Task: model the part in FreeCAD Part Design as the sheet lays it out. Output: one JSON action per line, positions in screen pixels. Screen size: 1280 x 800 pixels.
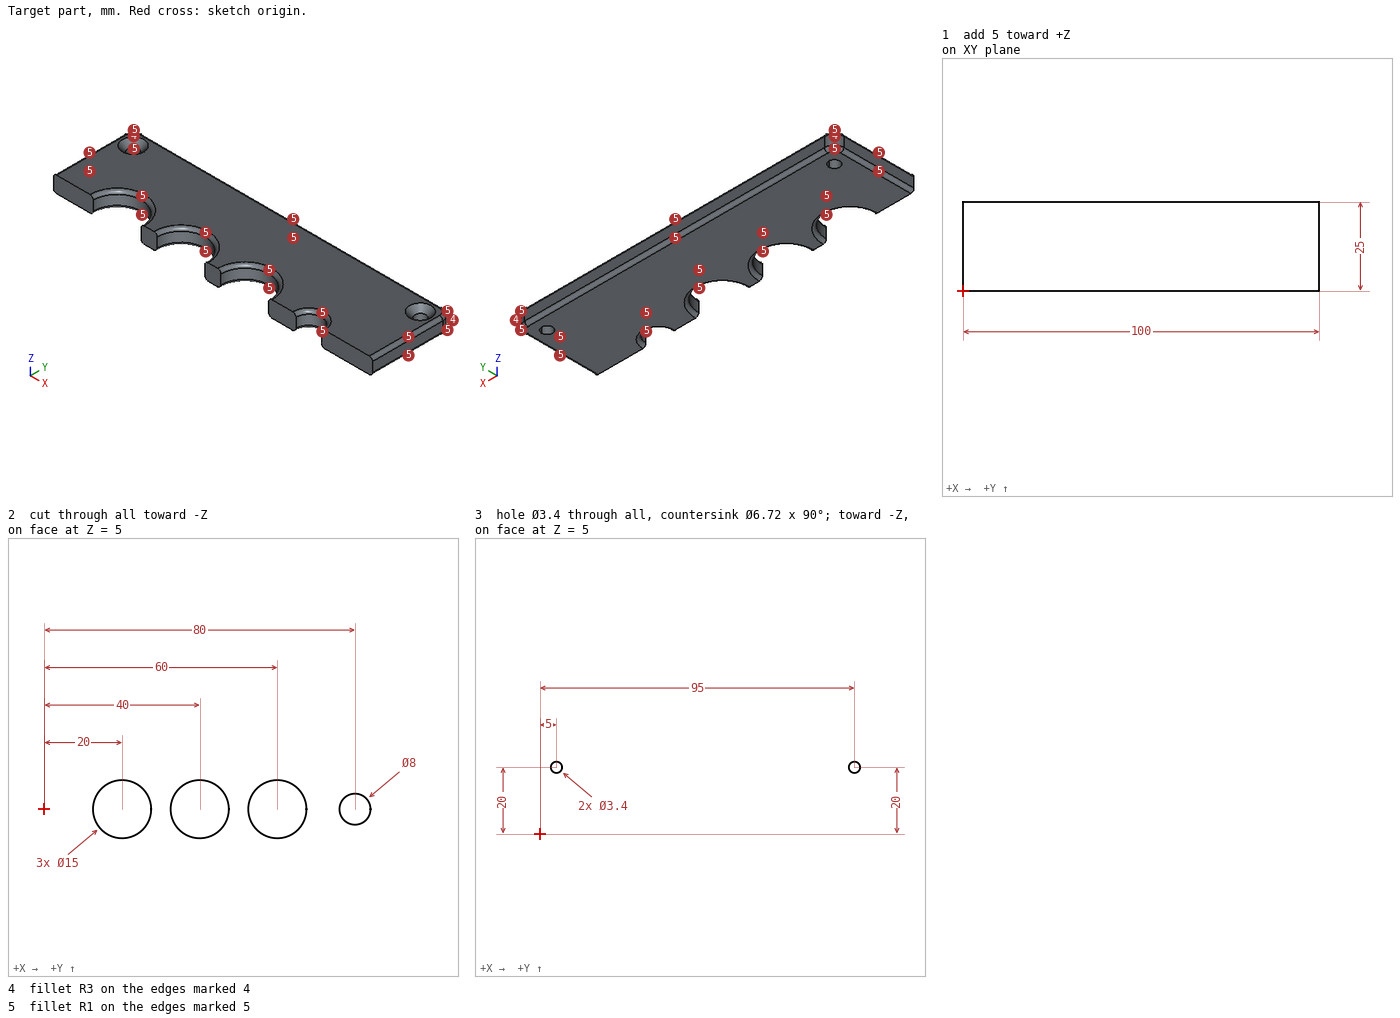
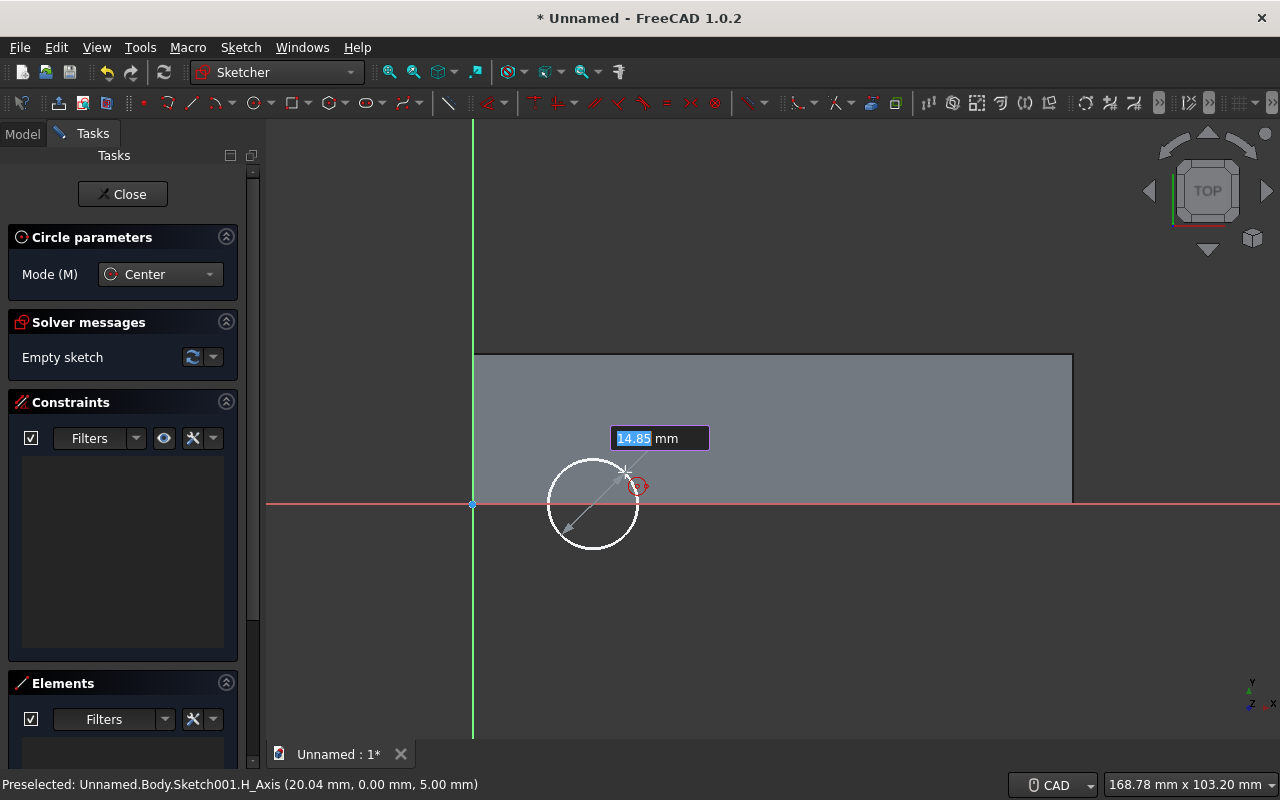
{"action": "type", "text": "15"}
{"action": "key", "text": "Return"}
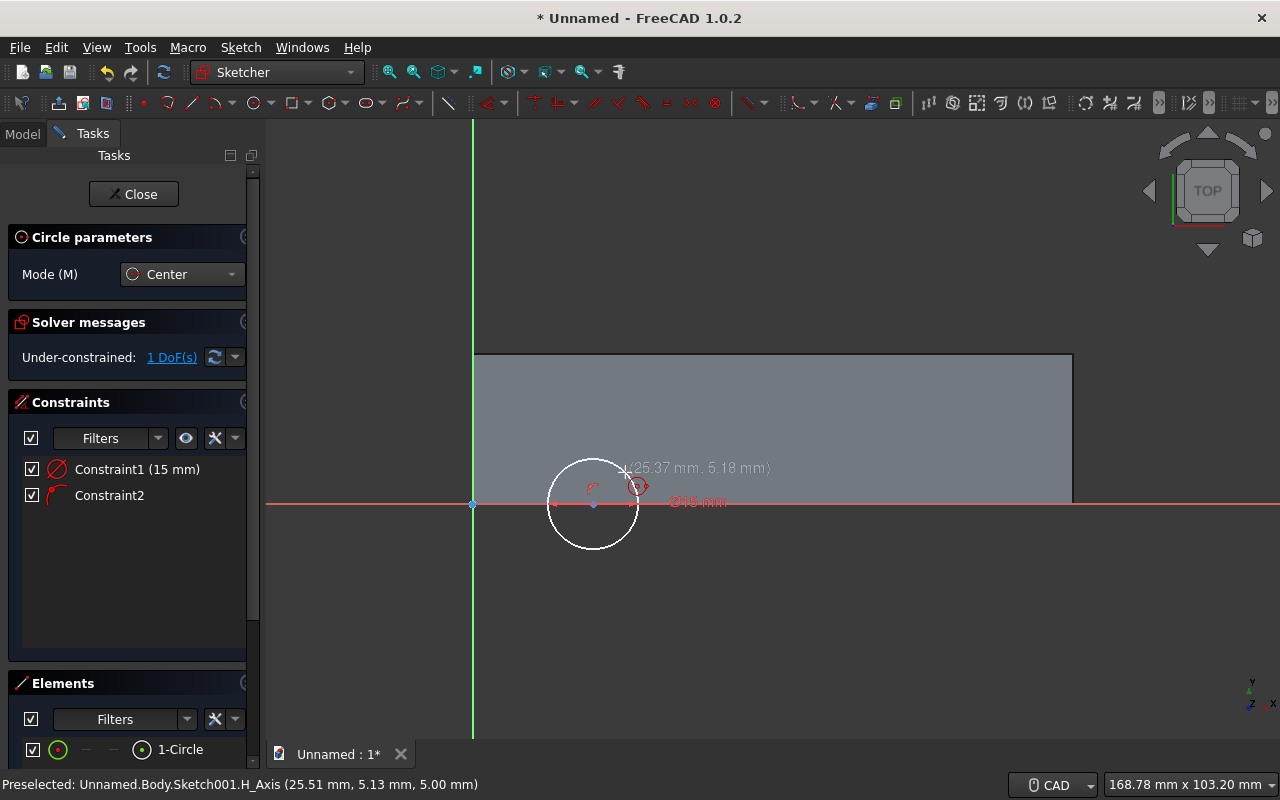
{"action": "left_click", "coordinate": [713, 504]}
{"action": "mouse_move", "coordinate": [745, 472]}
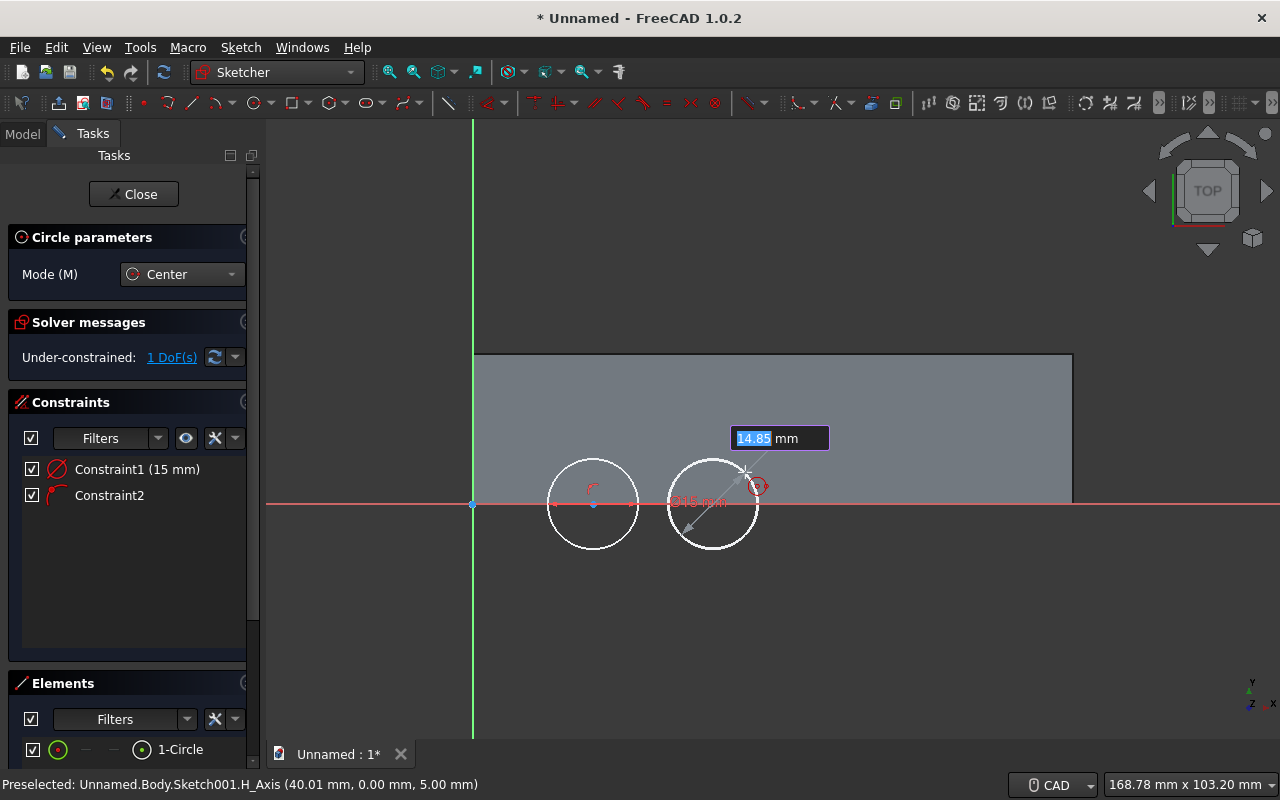
{"action": "type", "text": "15"}
{"action": "key", "text": "Return"}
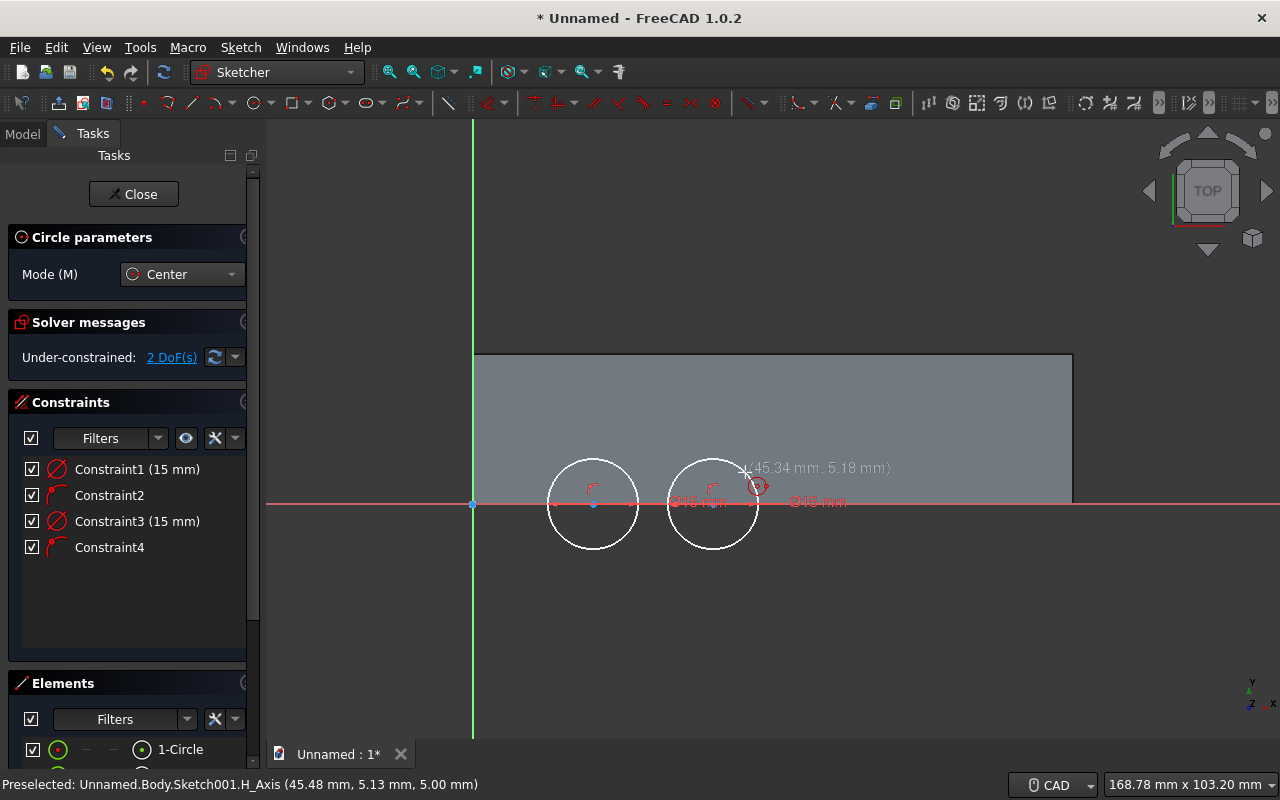
{"action": "left_click", "coordinate": [833, 504]}
{"action": "mouse_move", "coordinate": [865, 472]}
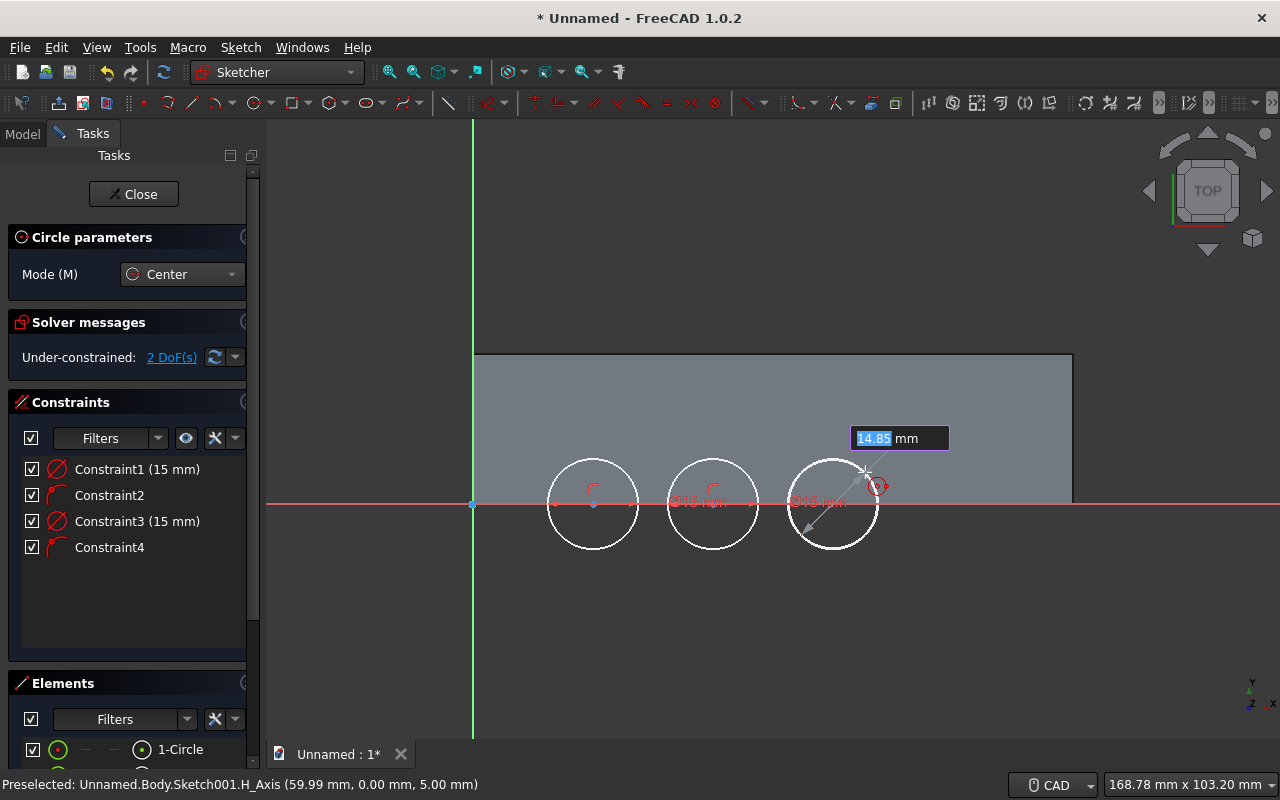
{"action": "type", "text": "15"}
{"action": "key", "text": "Return"}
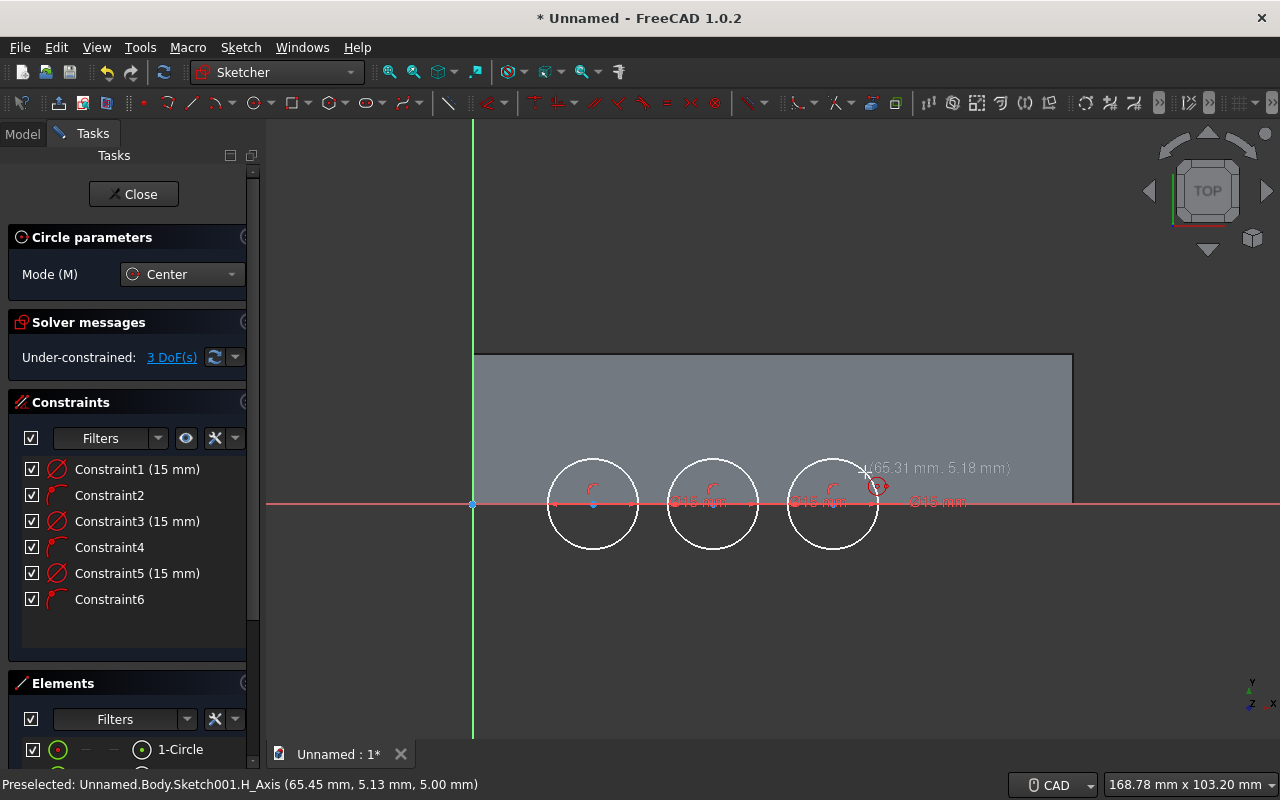
{"action": "left_click", "coordinate": [953, 504]}
{"action": "mouse_move", "coordinate": [970, 487]}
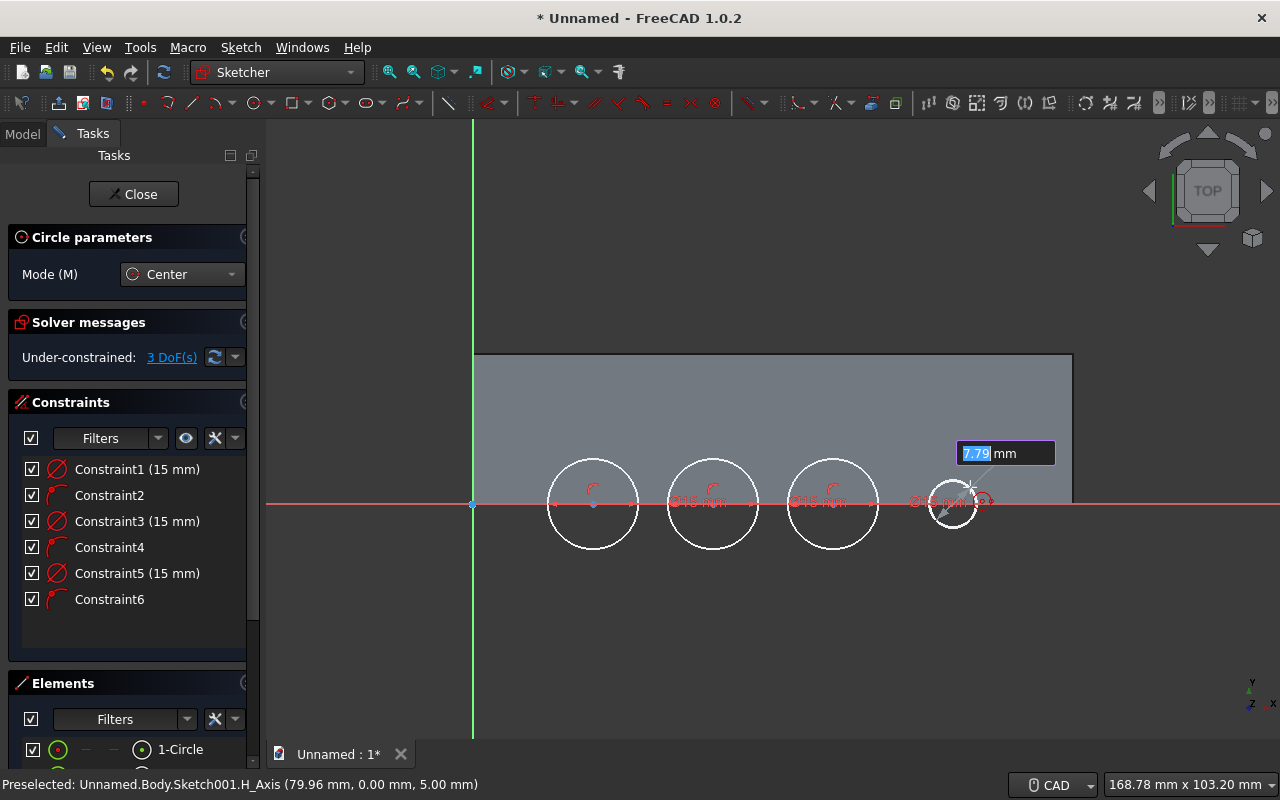
{"action": "type", "text": "8"}
{"action": "key", "text": "Return"}
{"action": "key", "text": "Escape"}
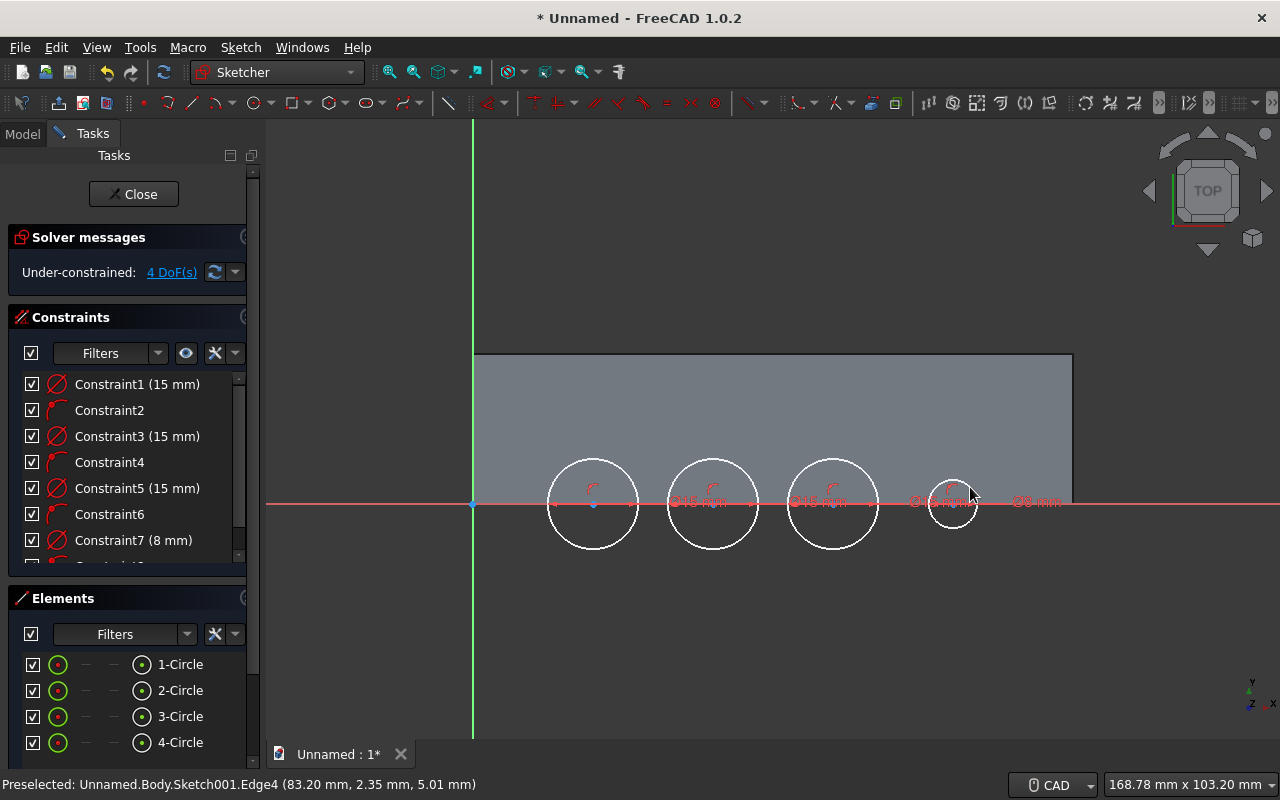
{"action": "left_click", "coordinate": [488, 104]}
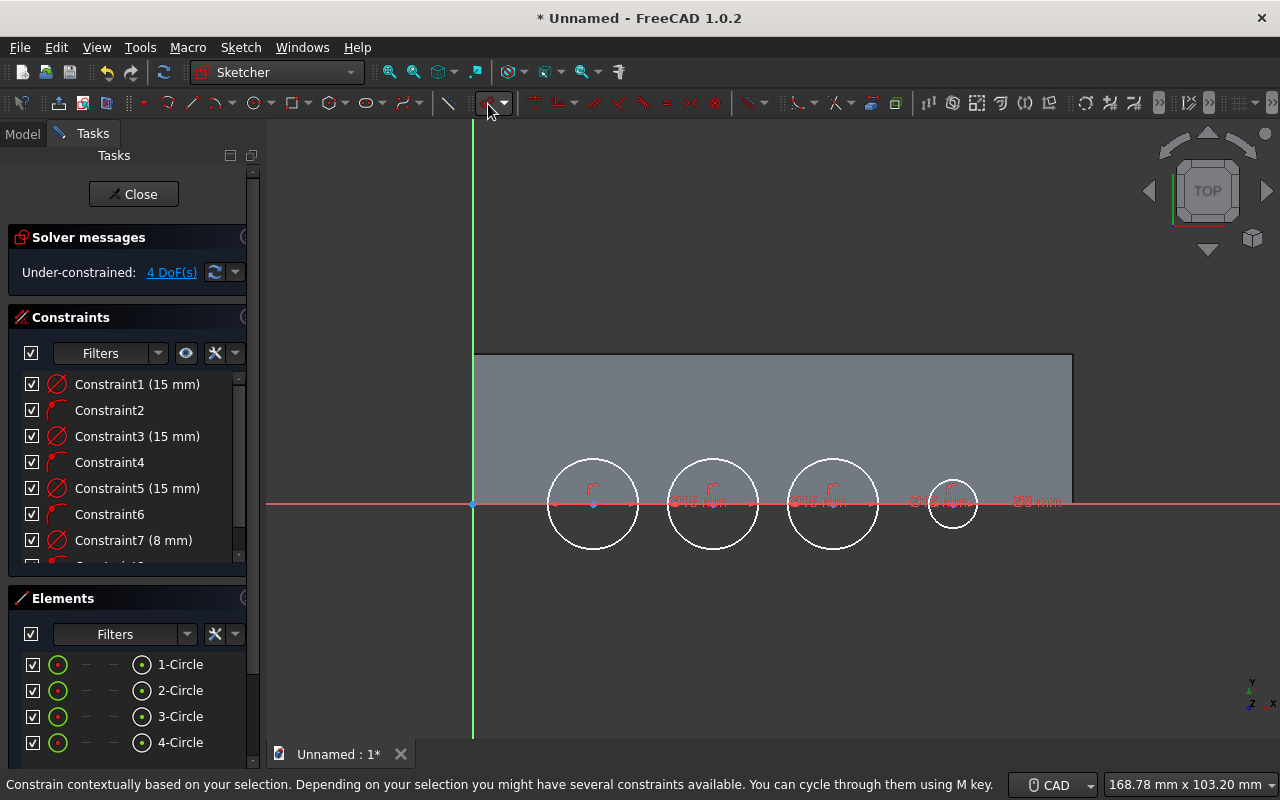
{"action": "left_click", "coordinate": [593, 504]}
{"action": "left_click", "coordinate": [533, 538]}